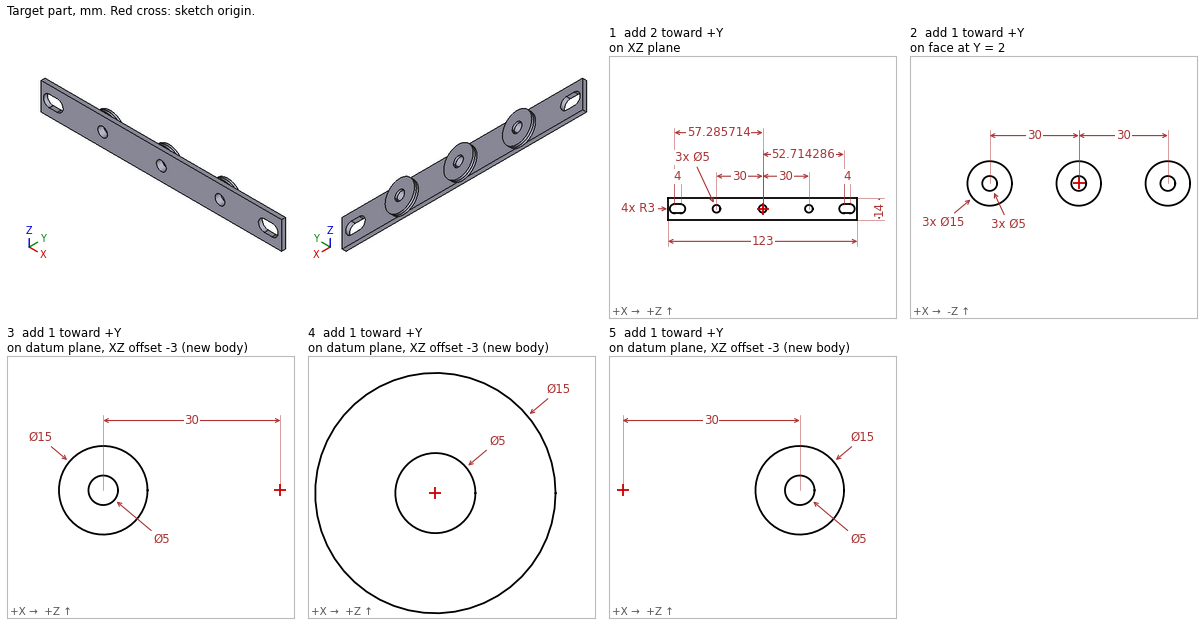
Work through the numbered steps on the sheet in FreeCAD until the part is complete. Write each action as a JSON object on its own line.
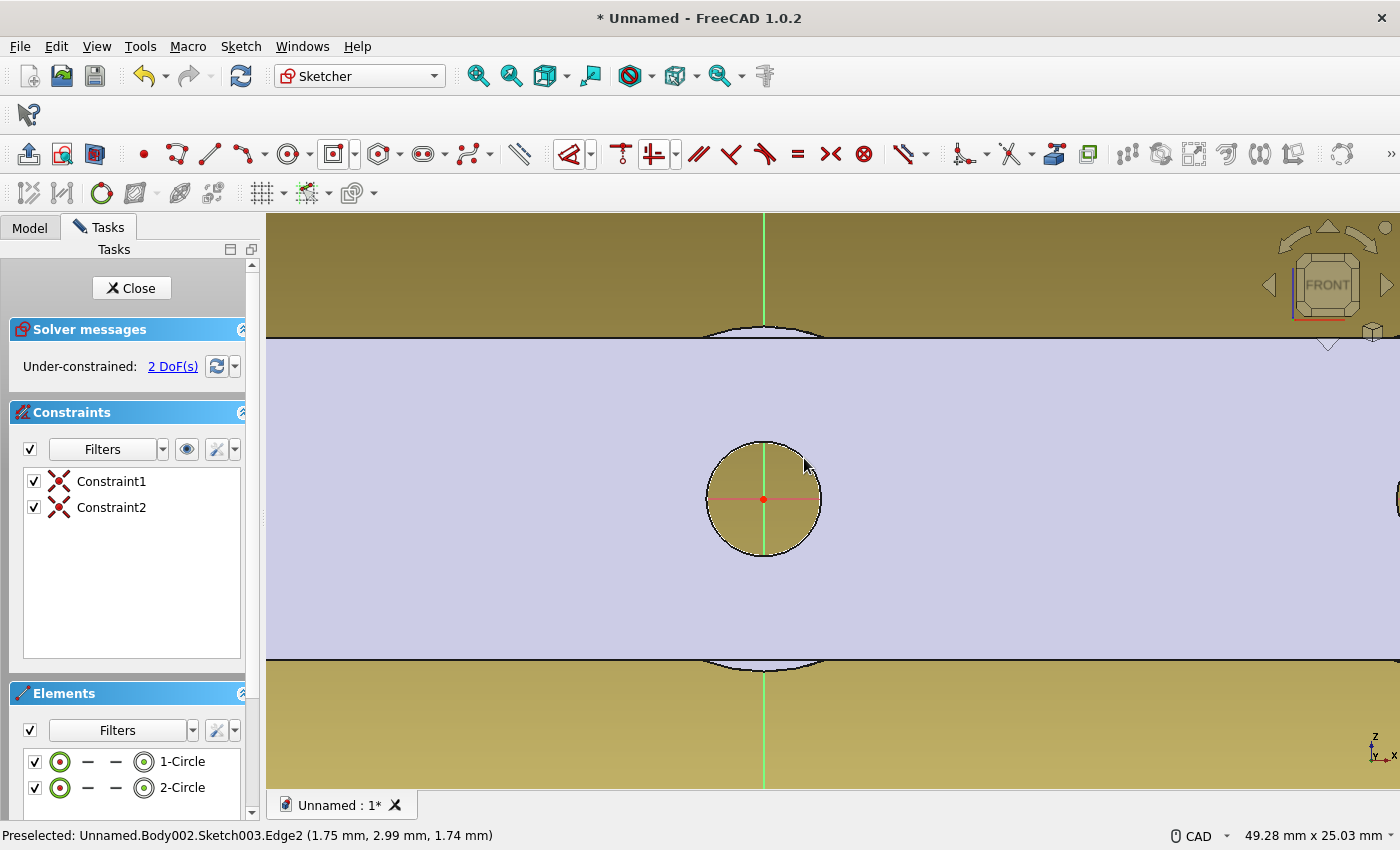
{"action": "left_click", "coordinate": [885, 377]}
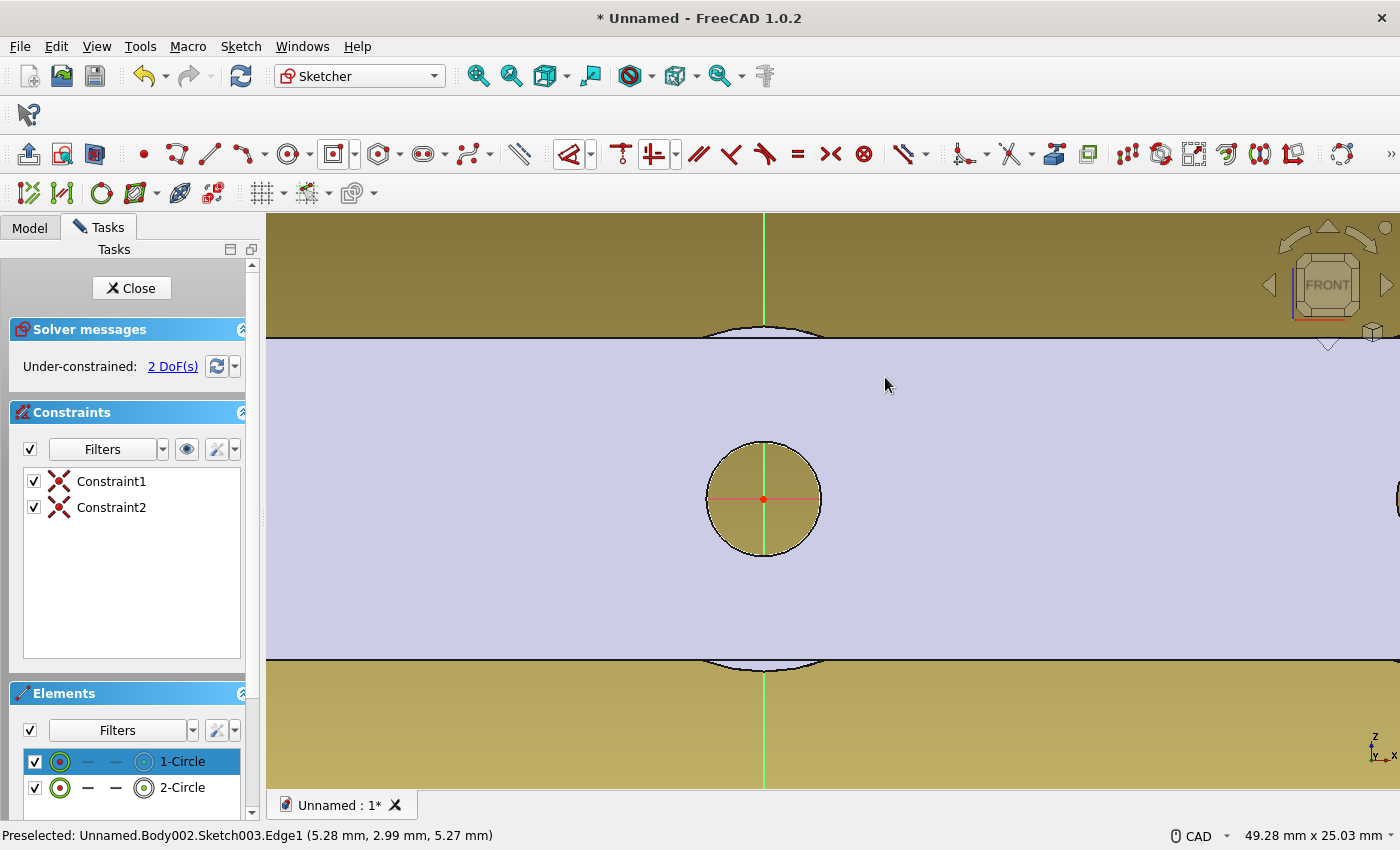
{"action": "left_click", "coordinate": [590, 154]}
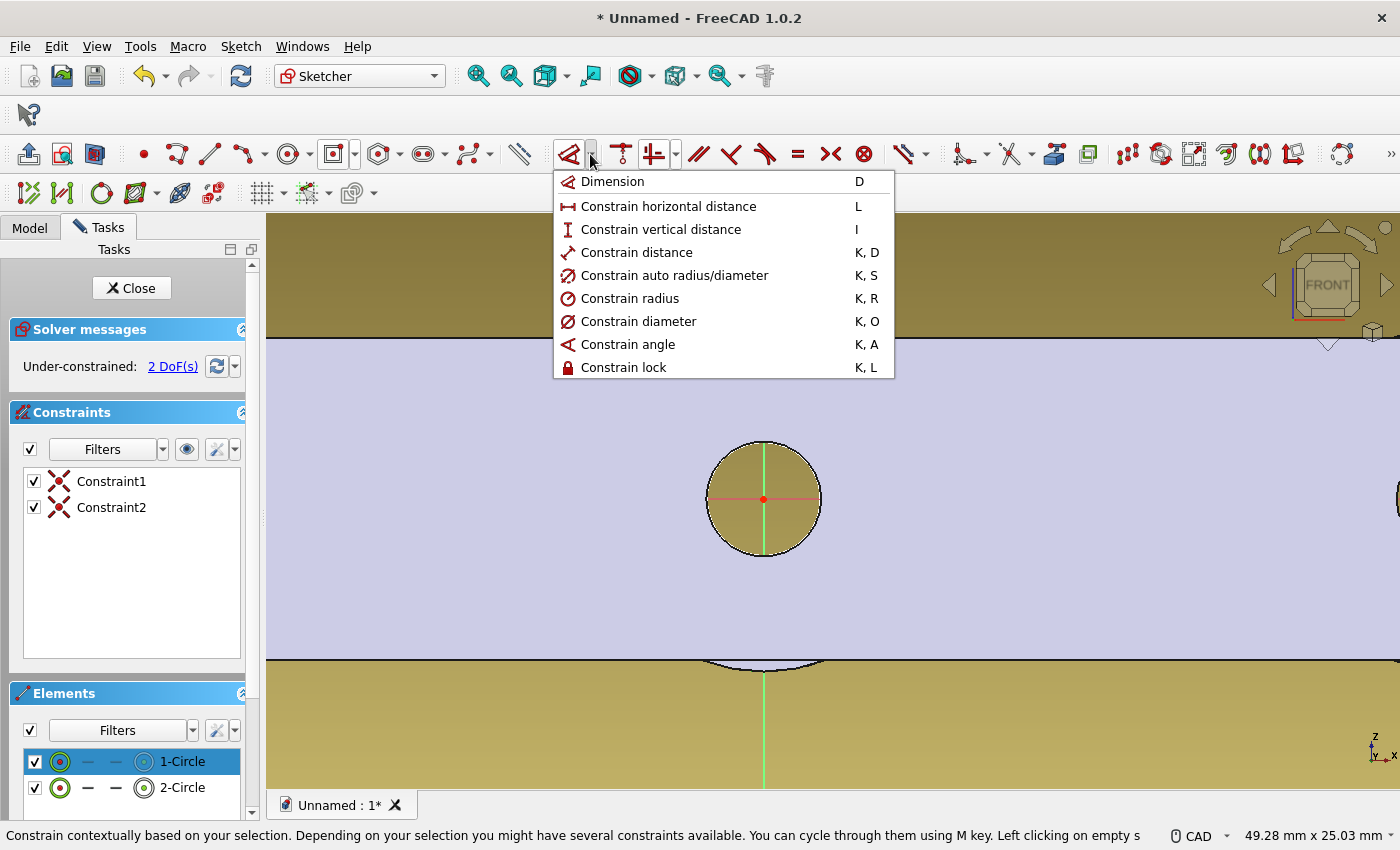
{"action": "left_click", "coordinate": [724, 322]}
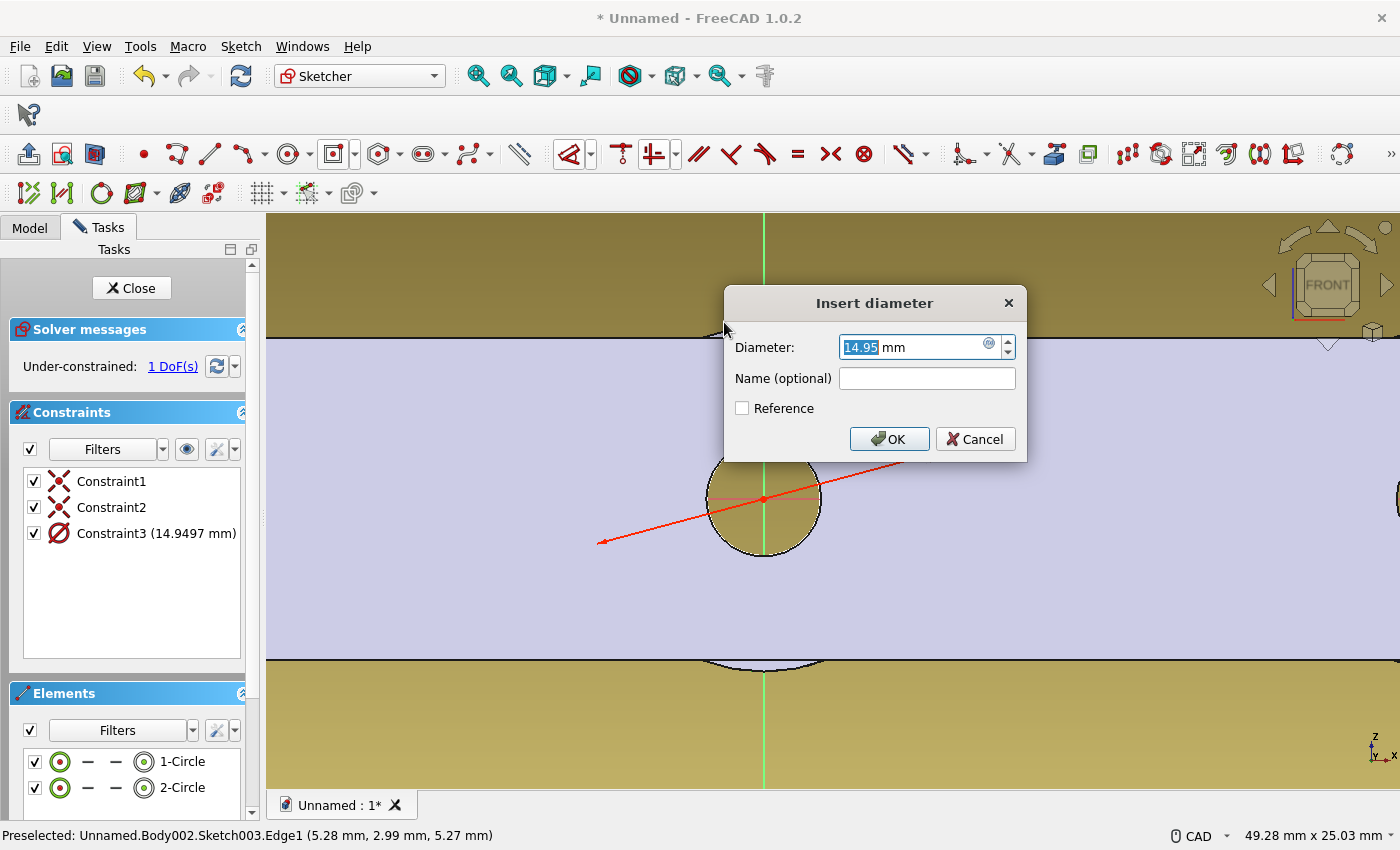
{"action": "type", "text": "15"}
{"action": "key", "text": "Return"}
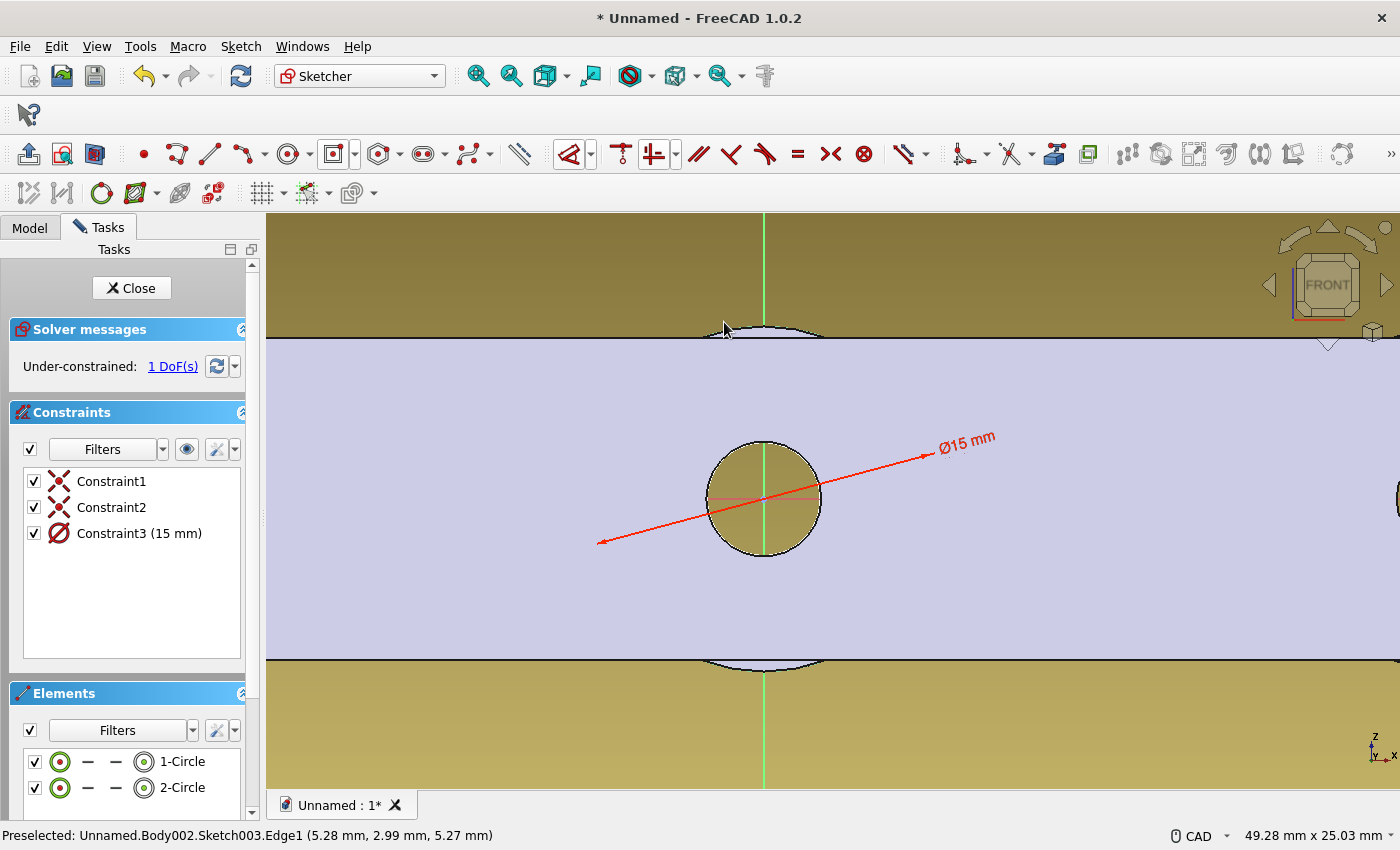
{"action": "left_click", "coordinate": [804, 459]}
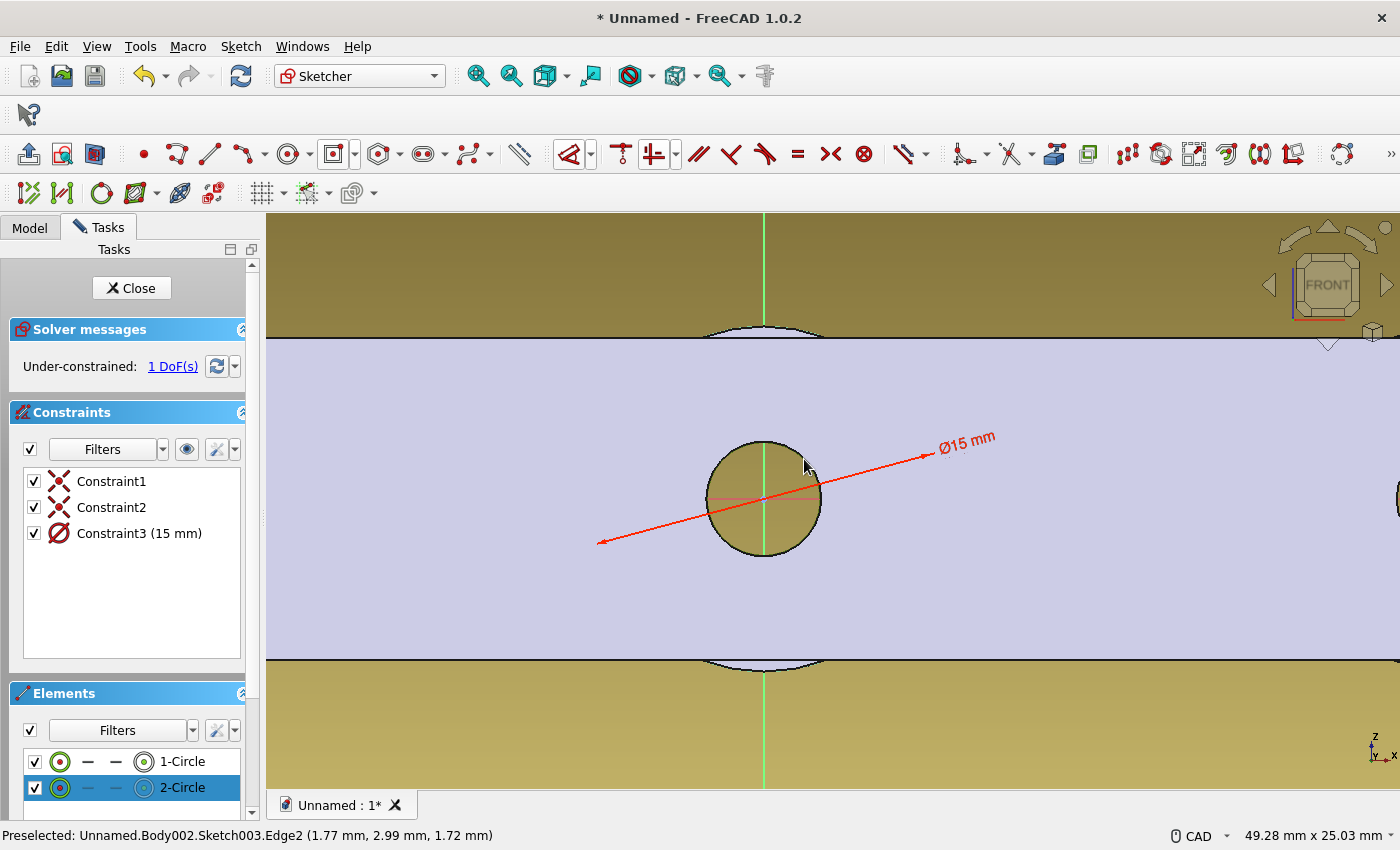
{"action": "key", "text": "k o"}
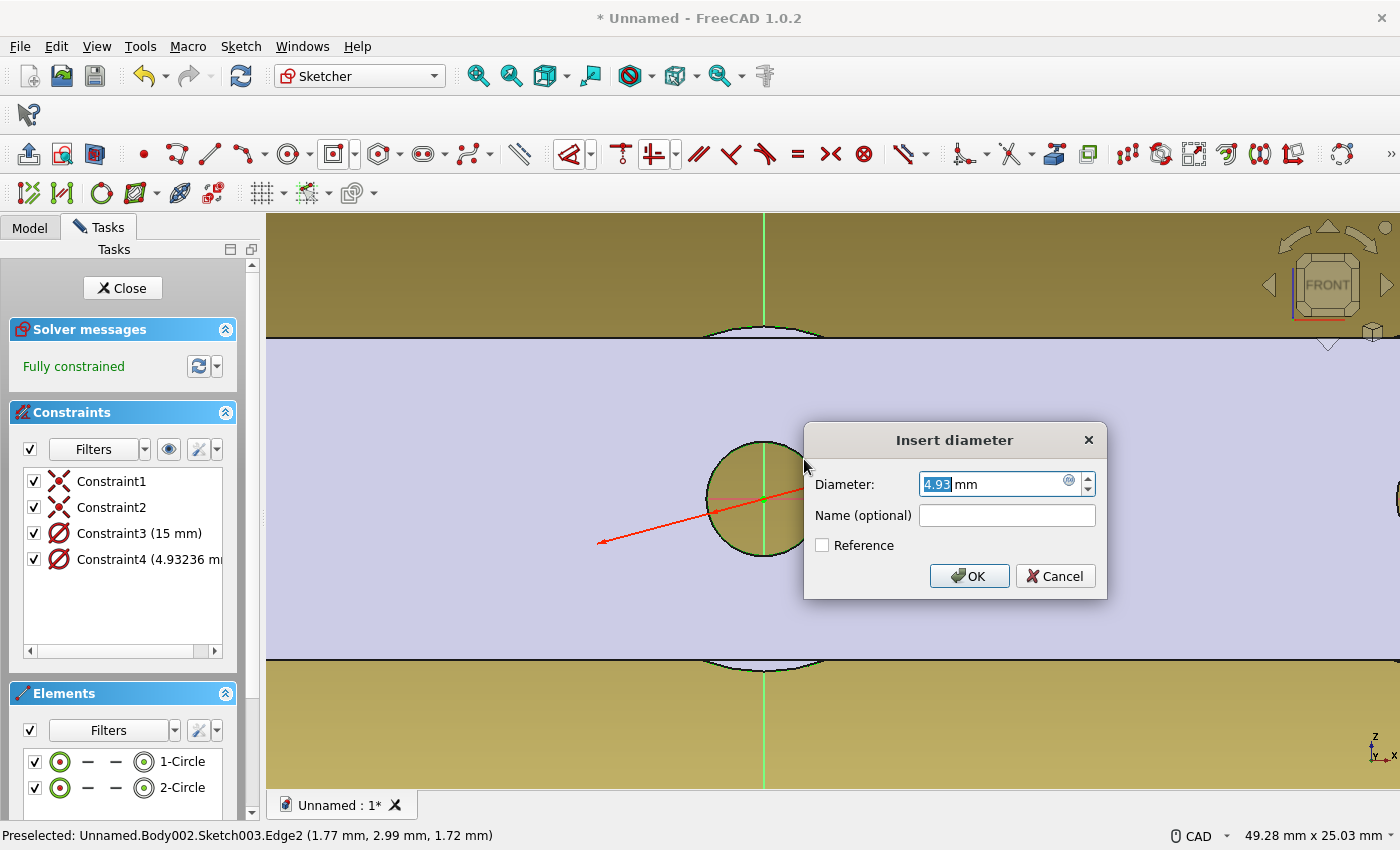
{"action": "type", "text": "5"}
{"action": "key", "text": "Return"}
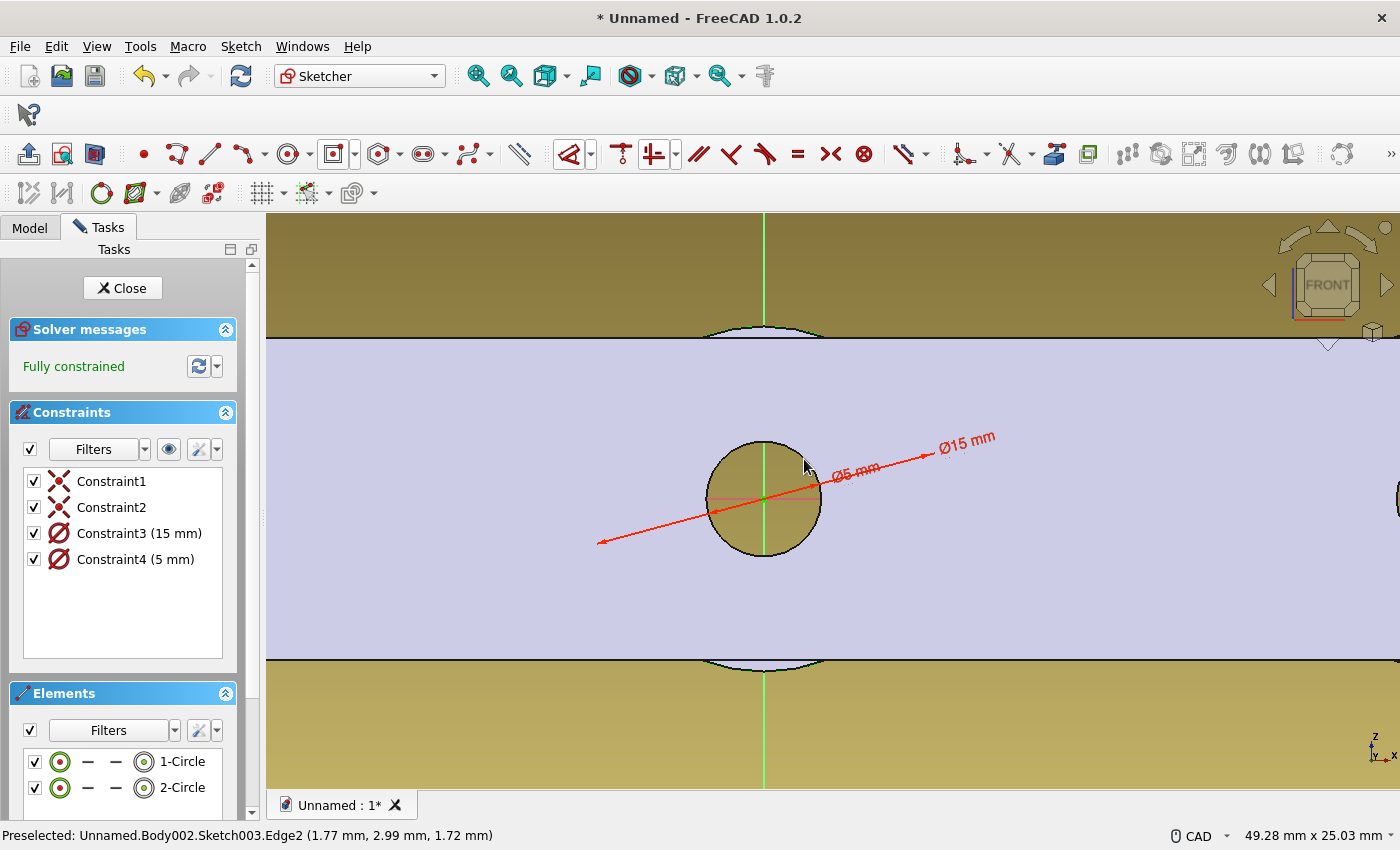
{"action": "left_click", "coordinate": [123, 288]}